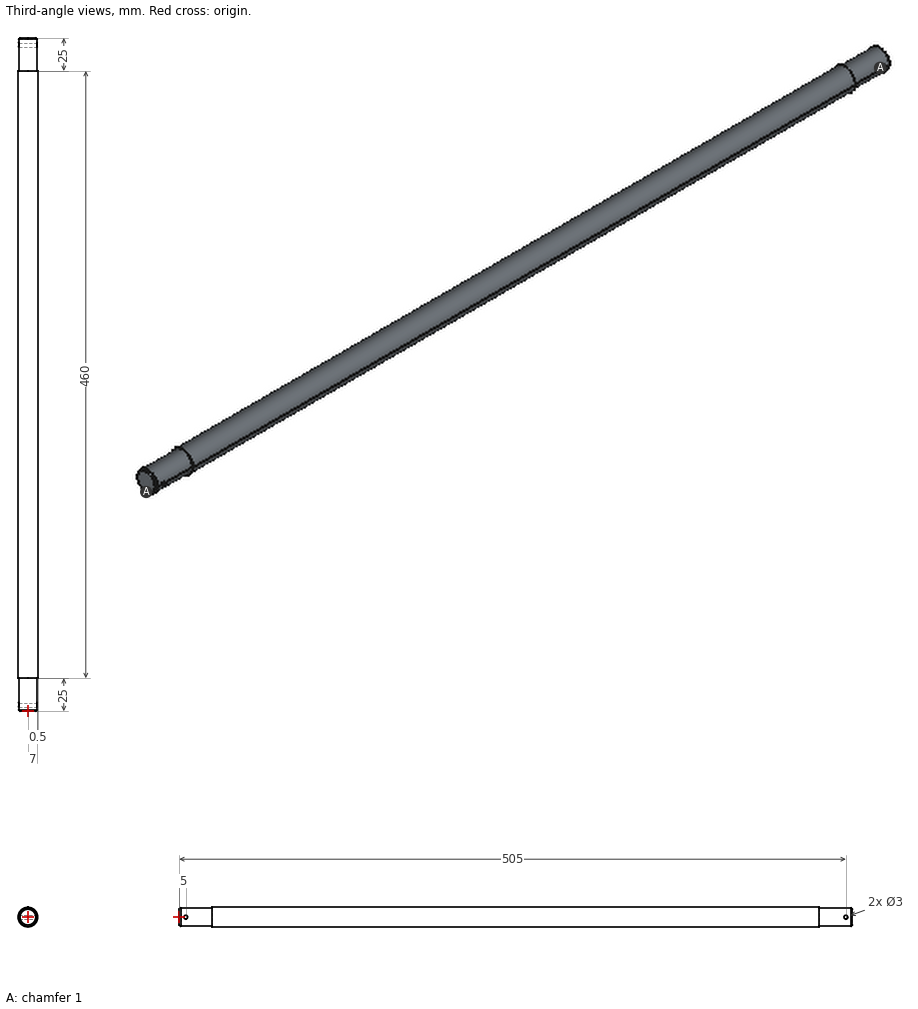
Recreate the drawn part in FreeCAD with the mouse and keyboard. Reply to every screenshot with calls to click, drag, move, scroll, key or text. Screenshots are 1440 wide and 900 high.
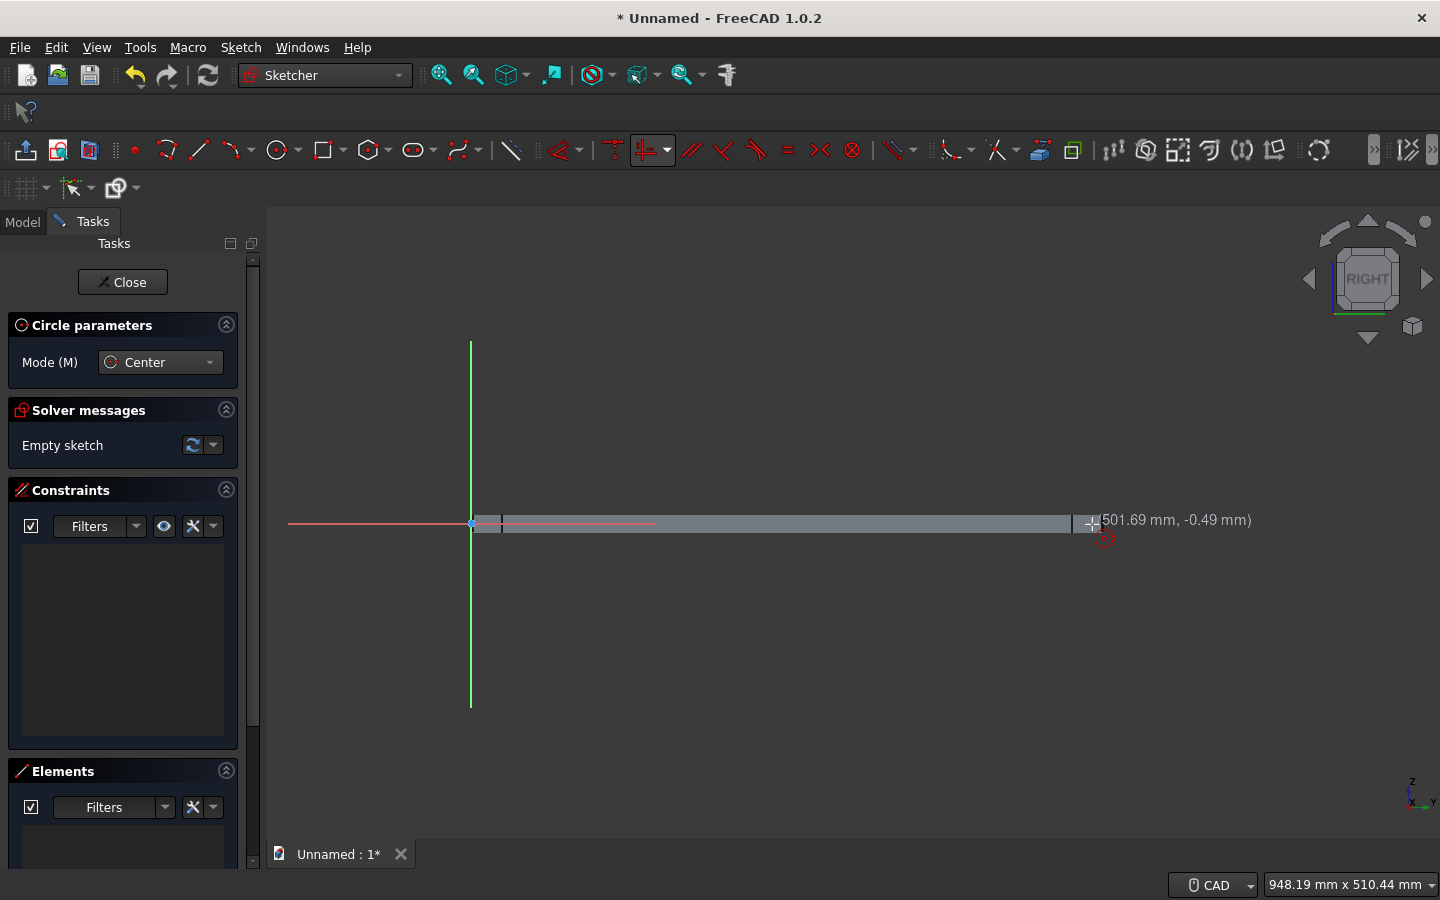
click(1097, 524)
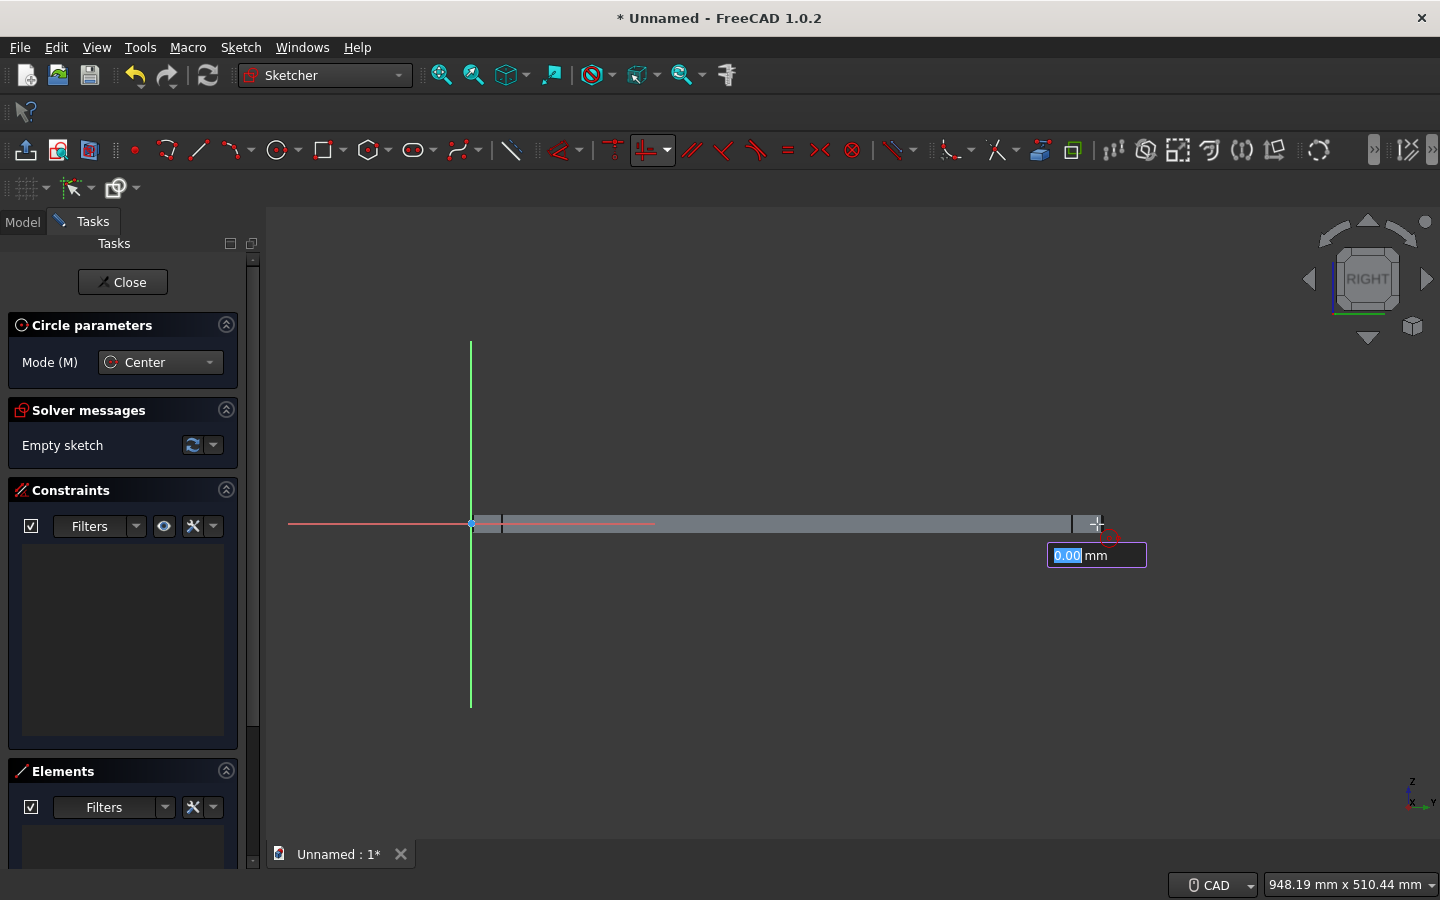
scroll(1096, 526, up, 12)
move(1090, 517)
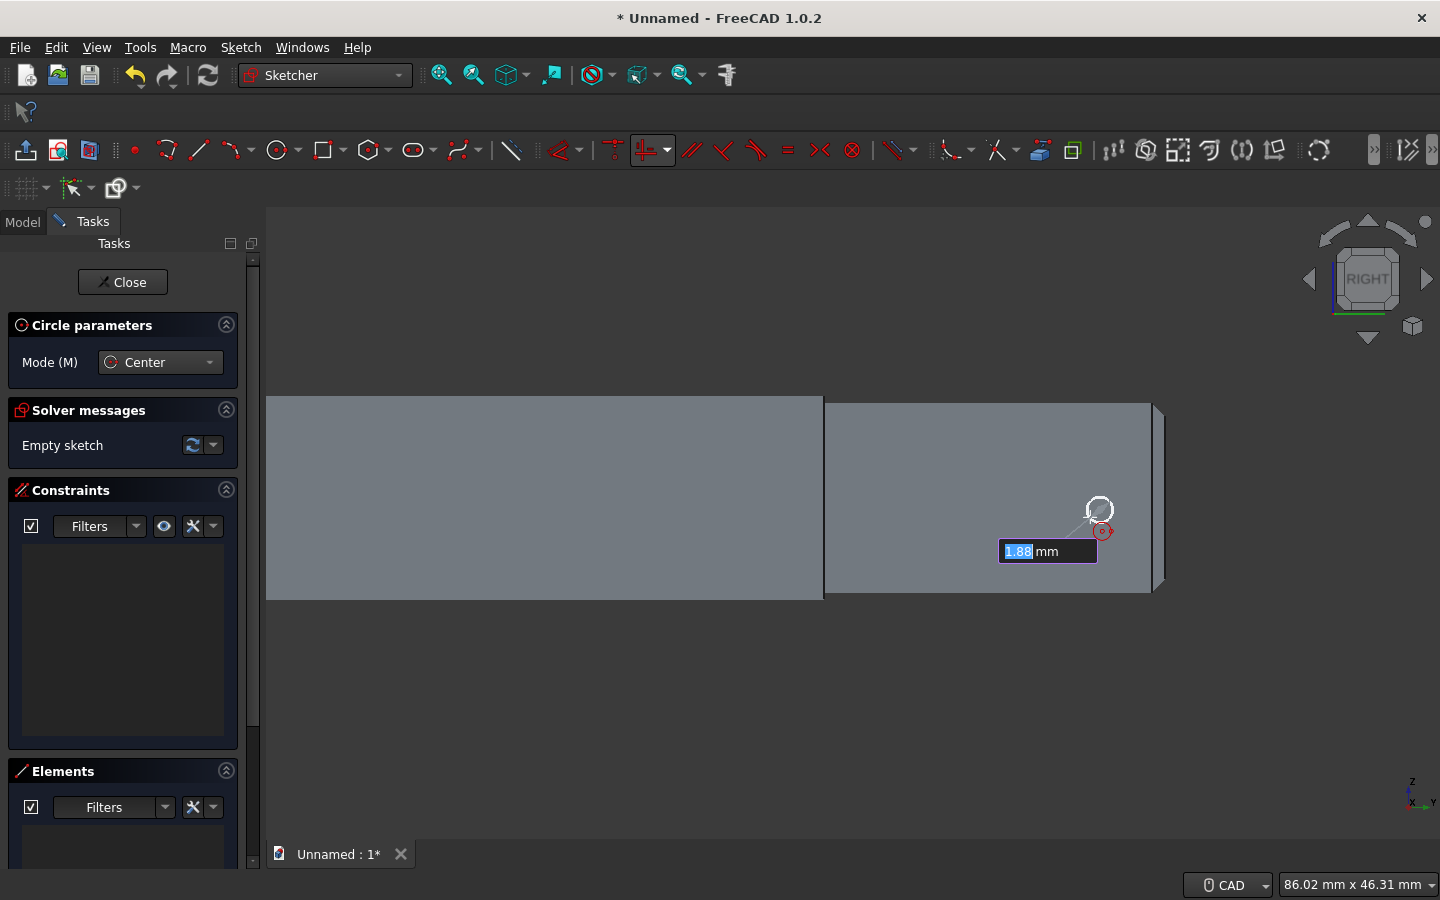
text(3)
key(Return)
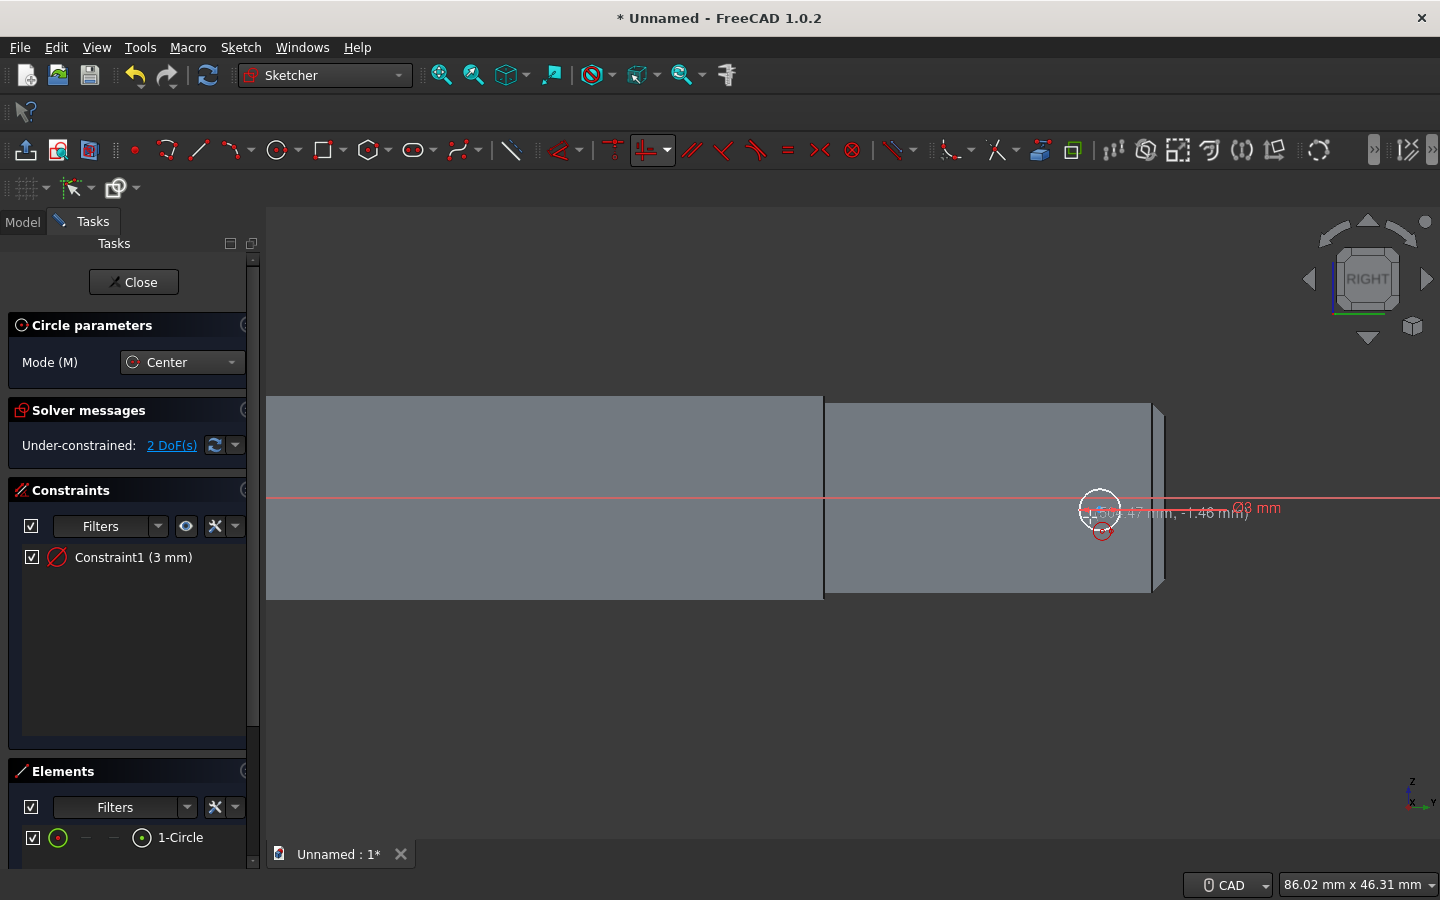
scroll(1096, 525, down, 12)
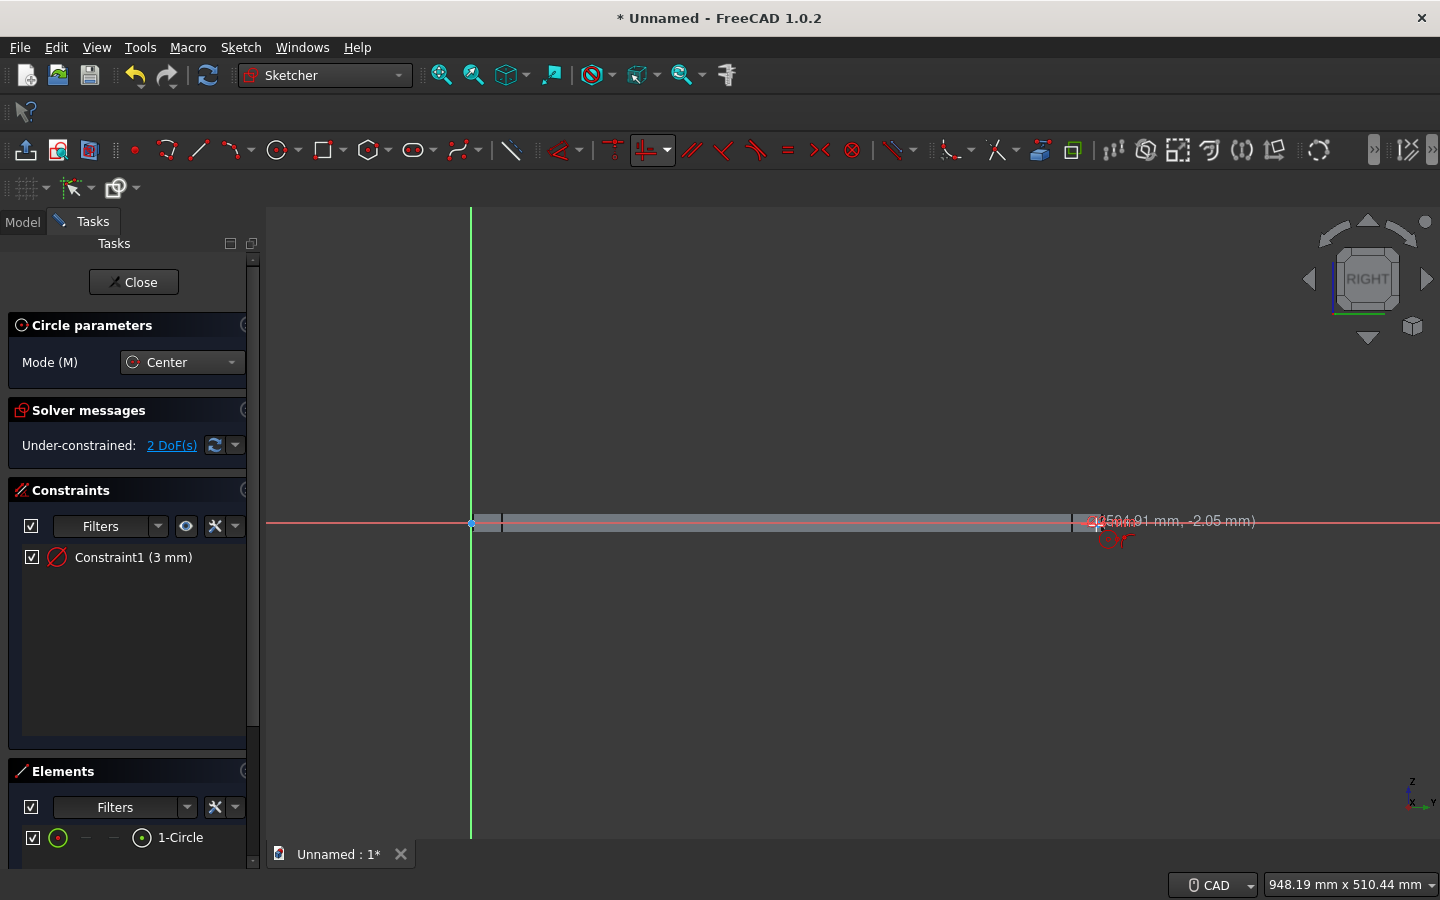
scroll(478, 523, up, 13)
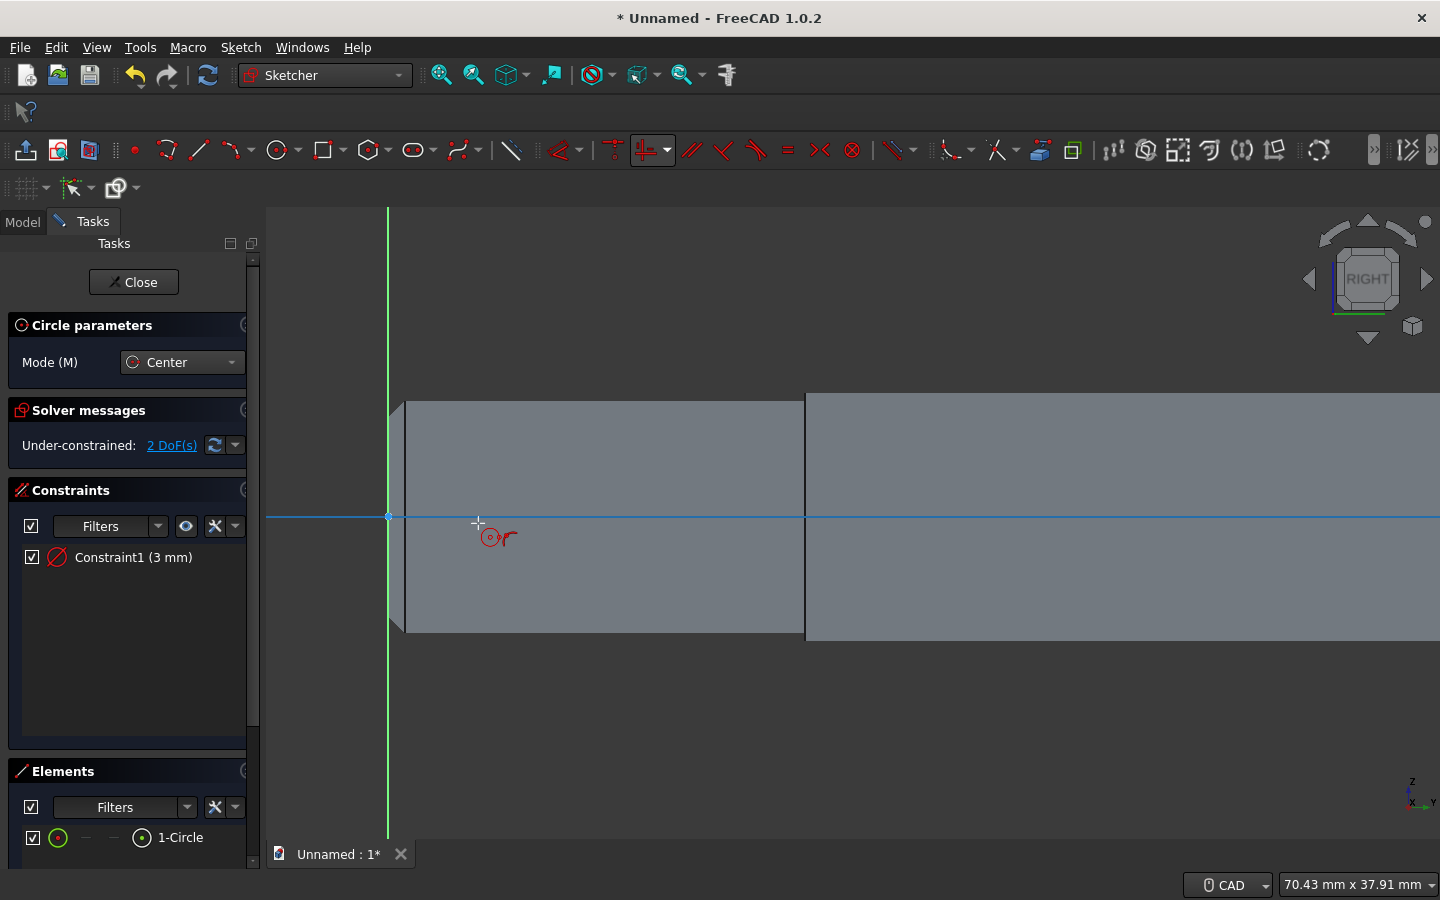
scroll(478, 523, down, 13)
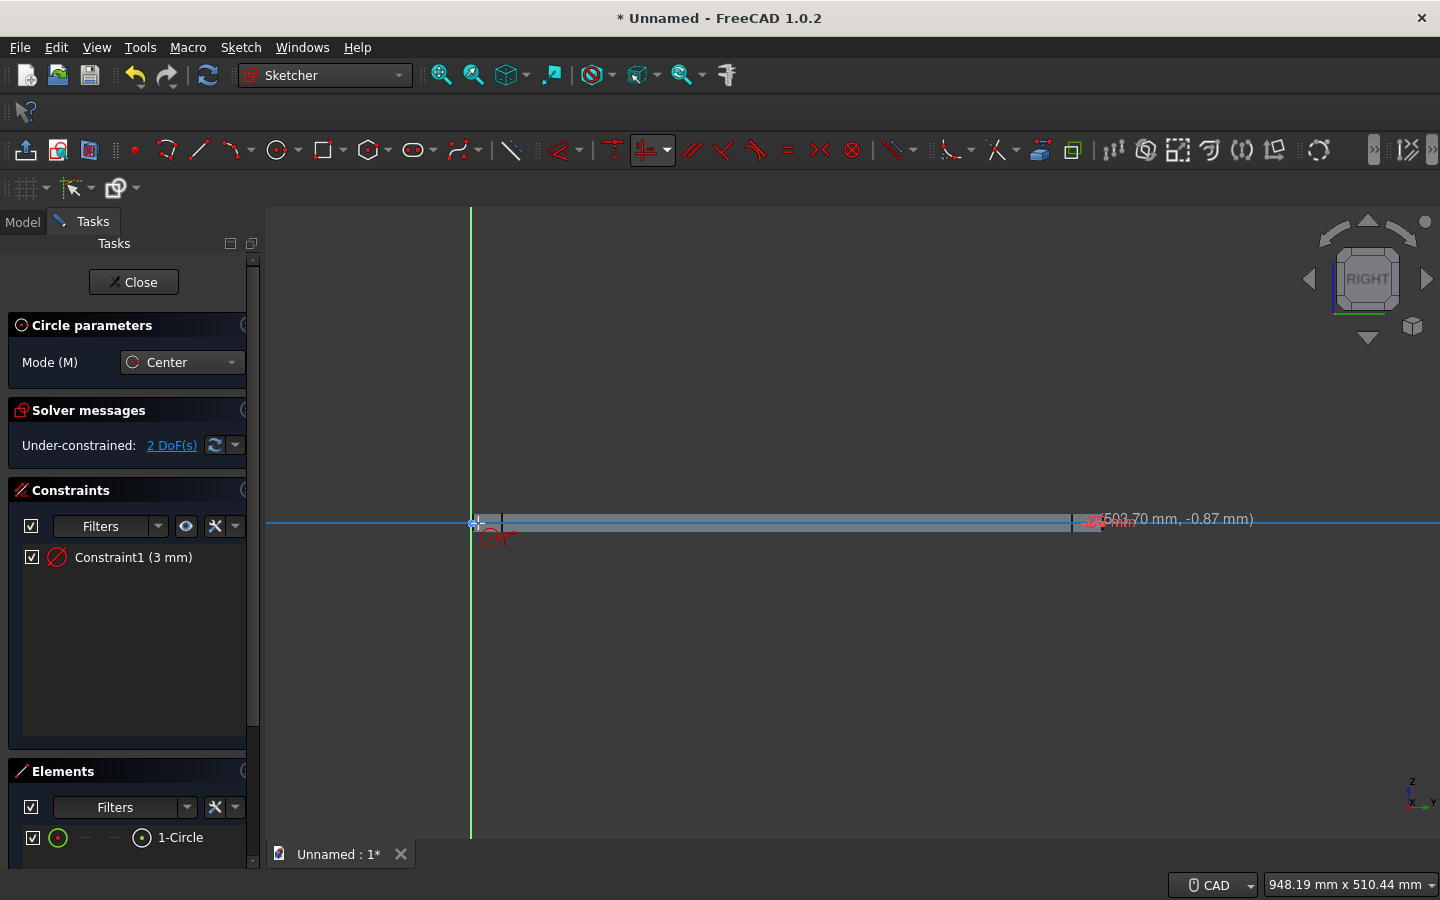
scroll(478, 523, up, 5)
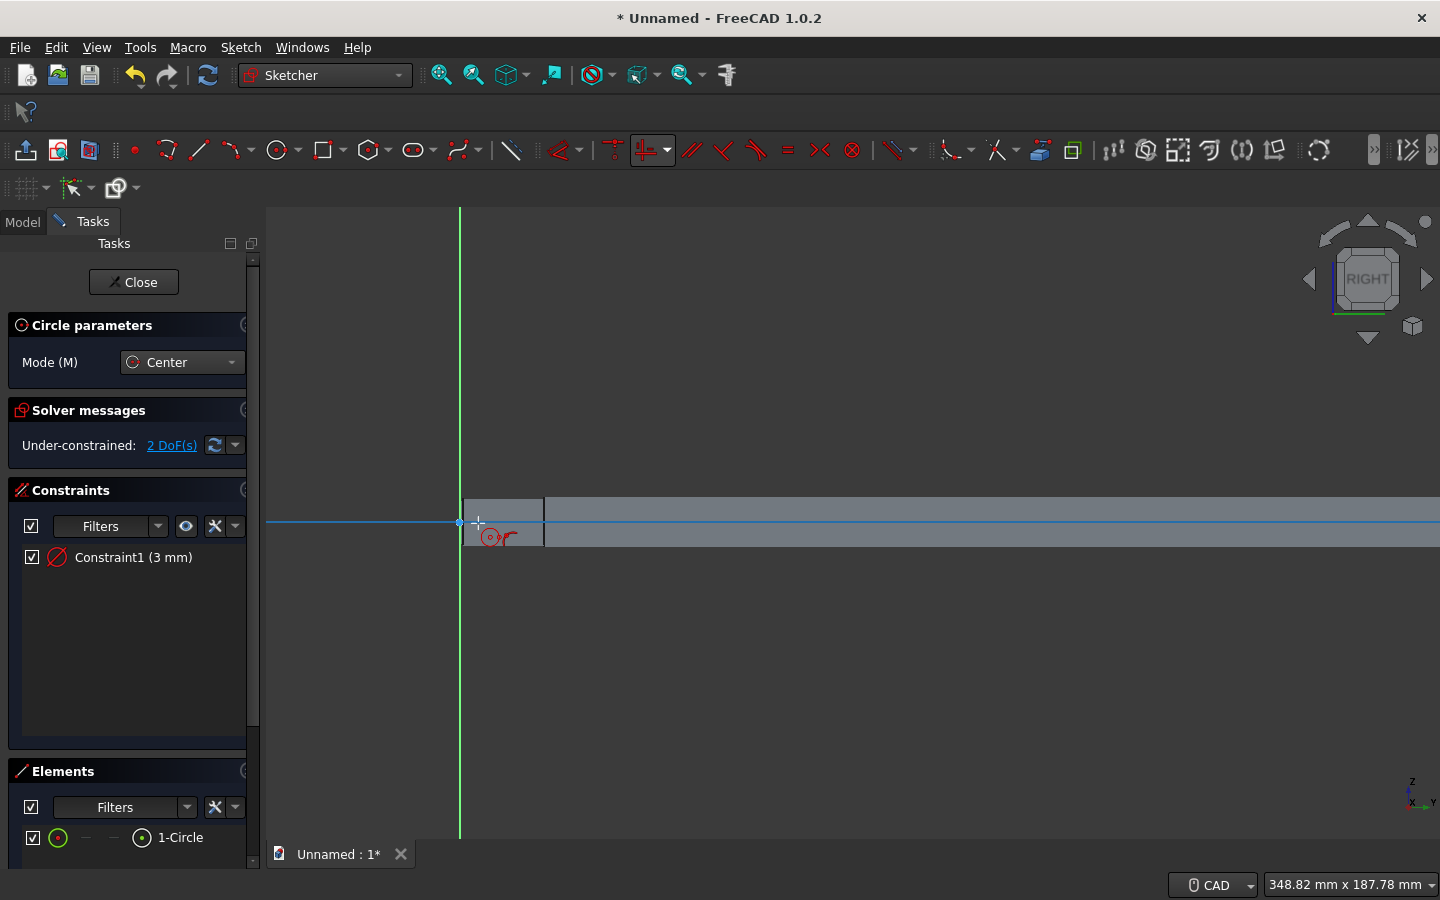
click(477, 522)